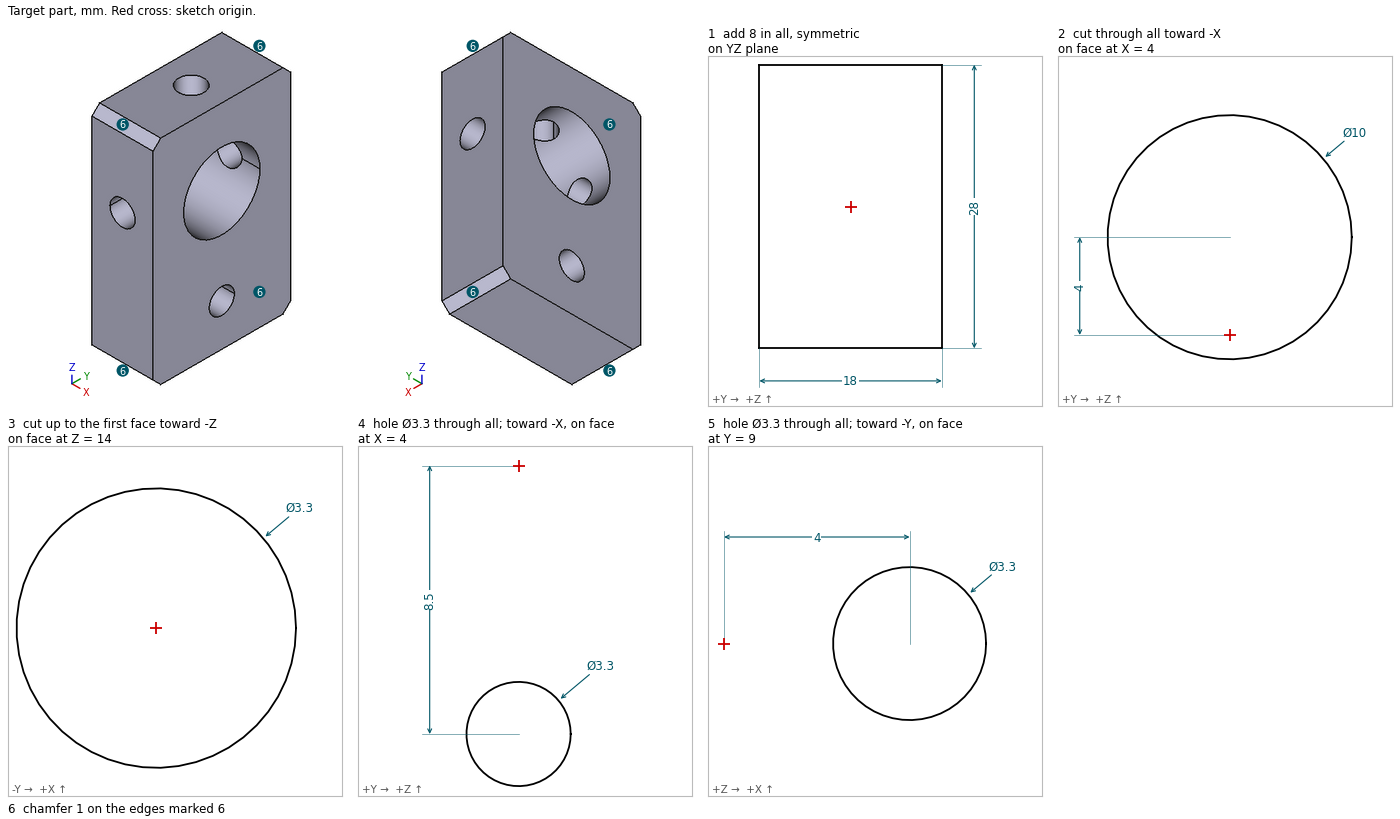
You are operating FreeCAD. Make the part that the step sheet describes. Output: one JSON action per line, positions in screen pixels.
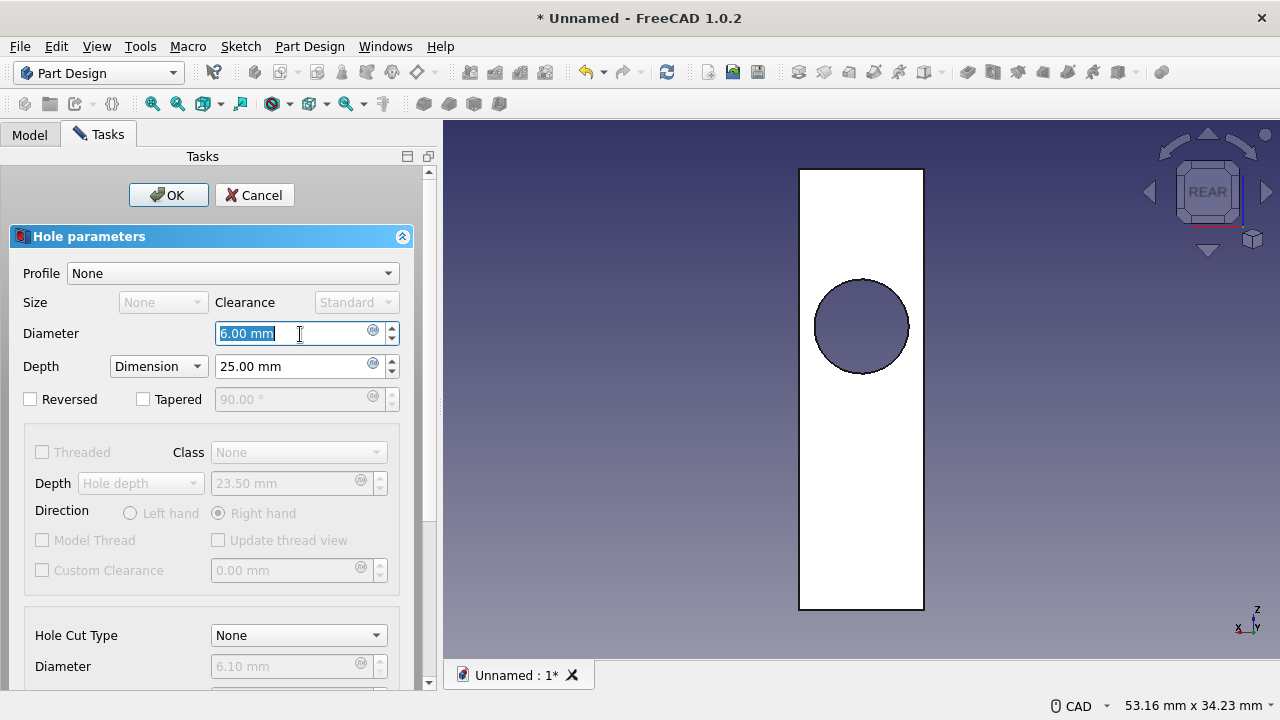
{"action": "type", "text": "3.3"}
{"action": "key", "text": "Tab"}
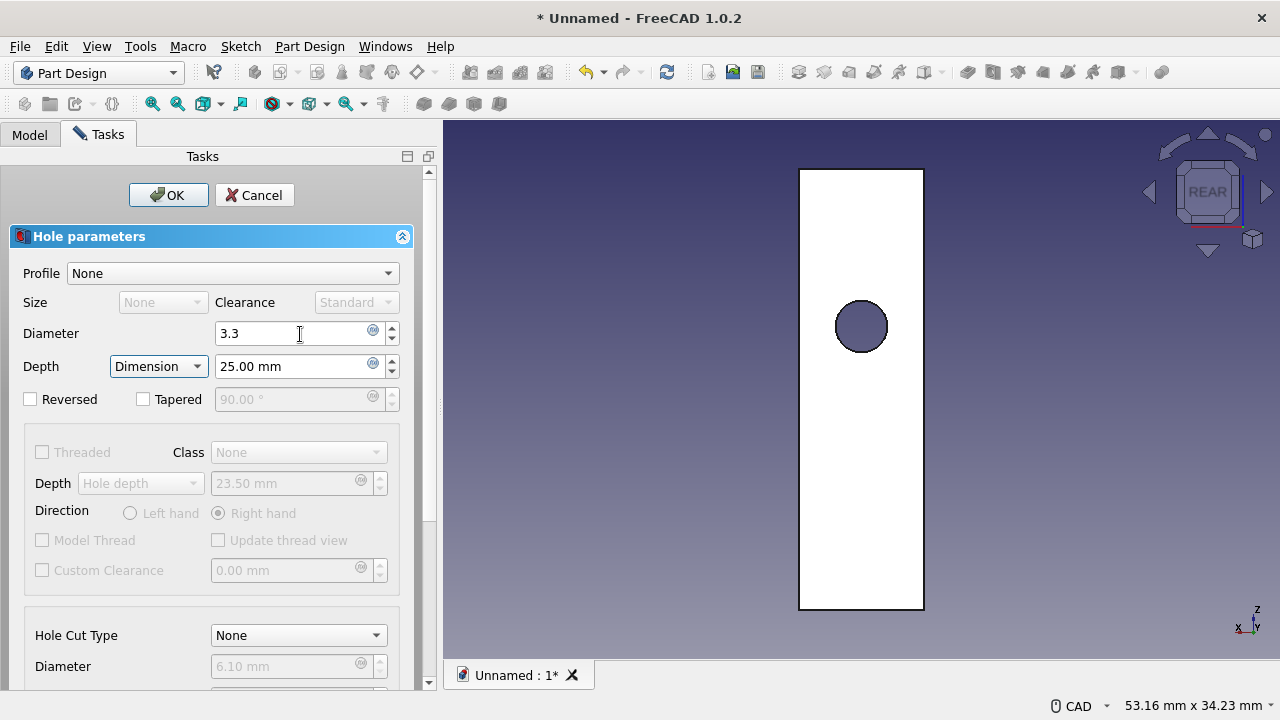
{"action": "left_click", "coordinate": [160, 366]}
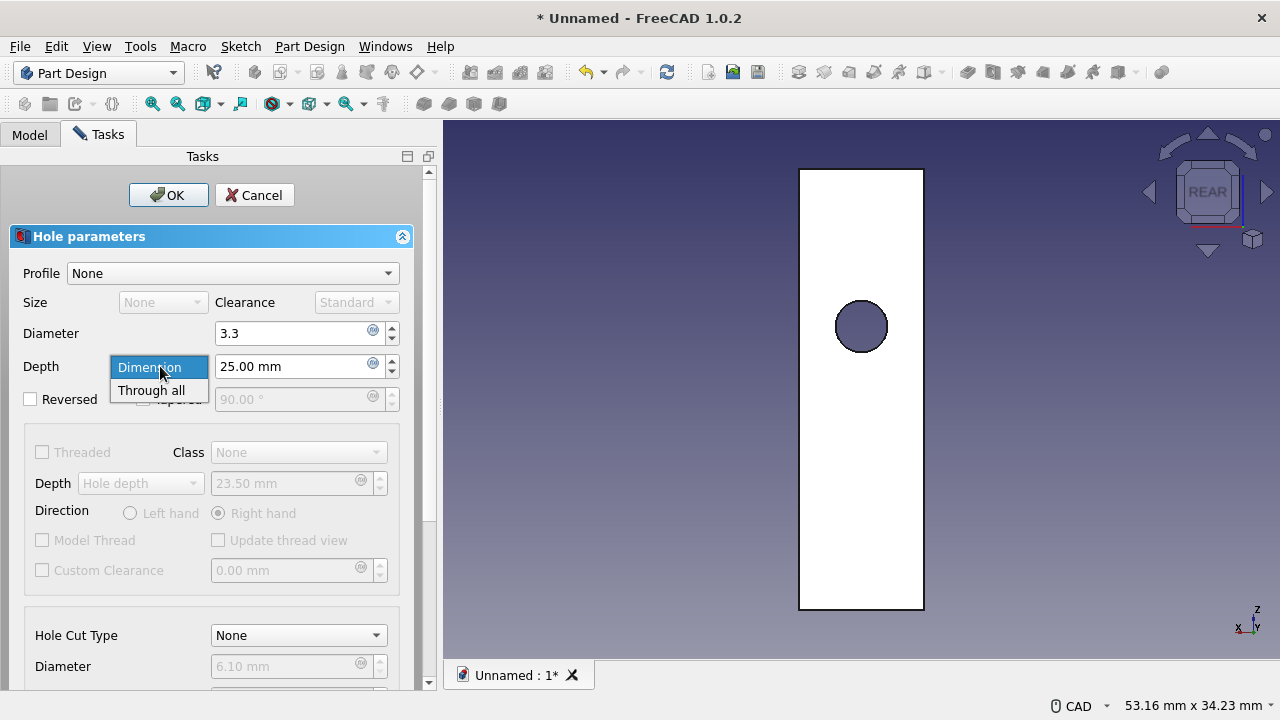
{"action": "left_click", "coordinate": [158, 390]}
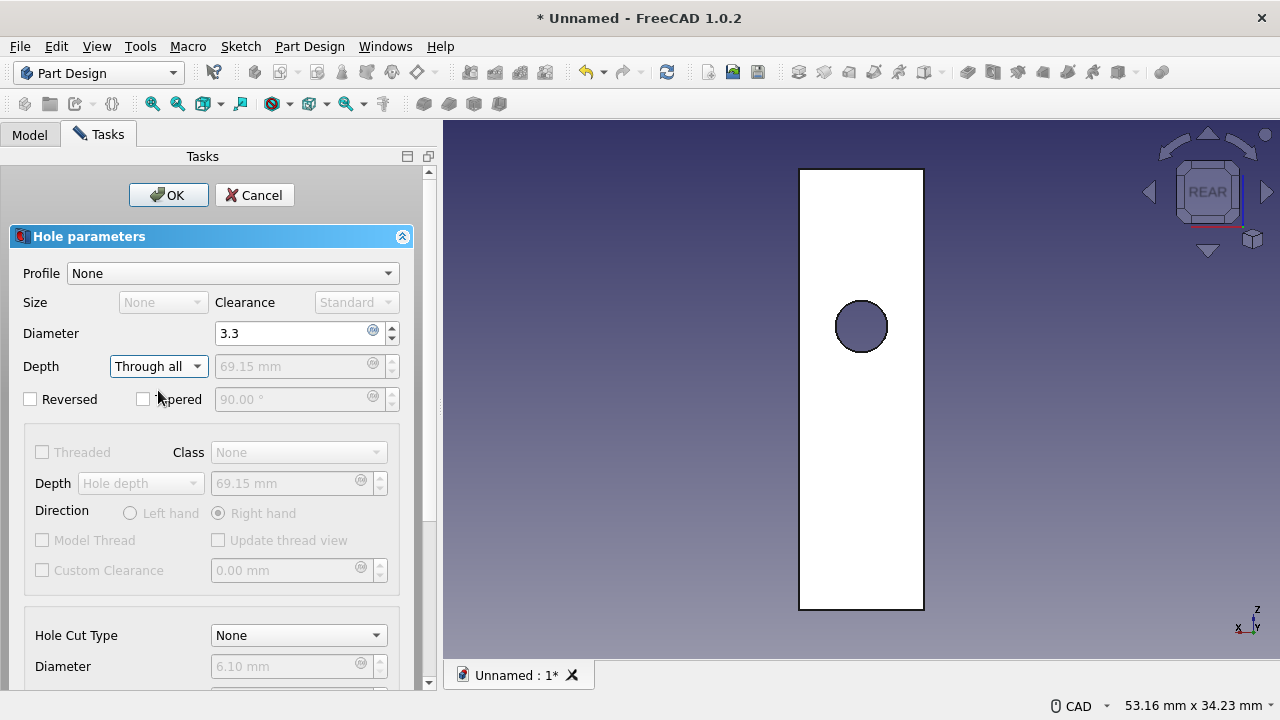
{"action": "left_click", "coordinate": [169, 195]}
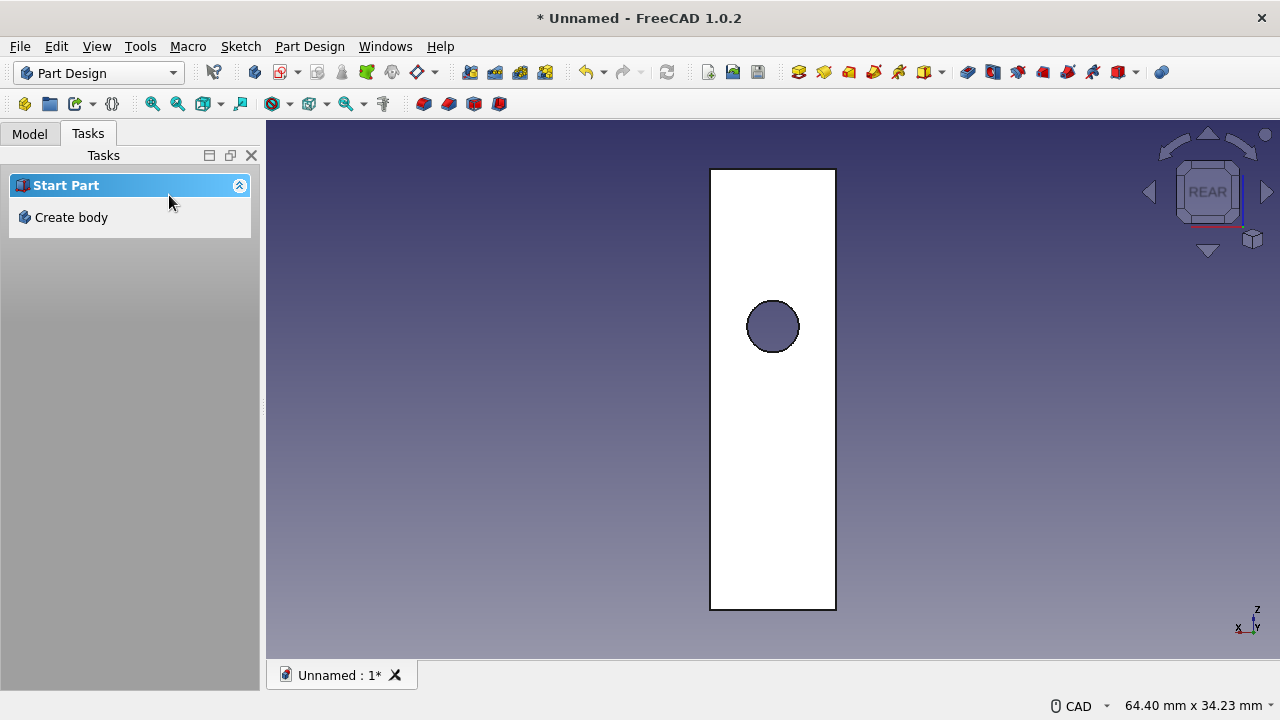
{"action": "left_click", "coordinate": [773, 168]}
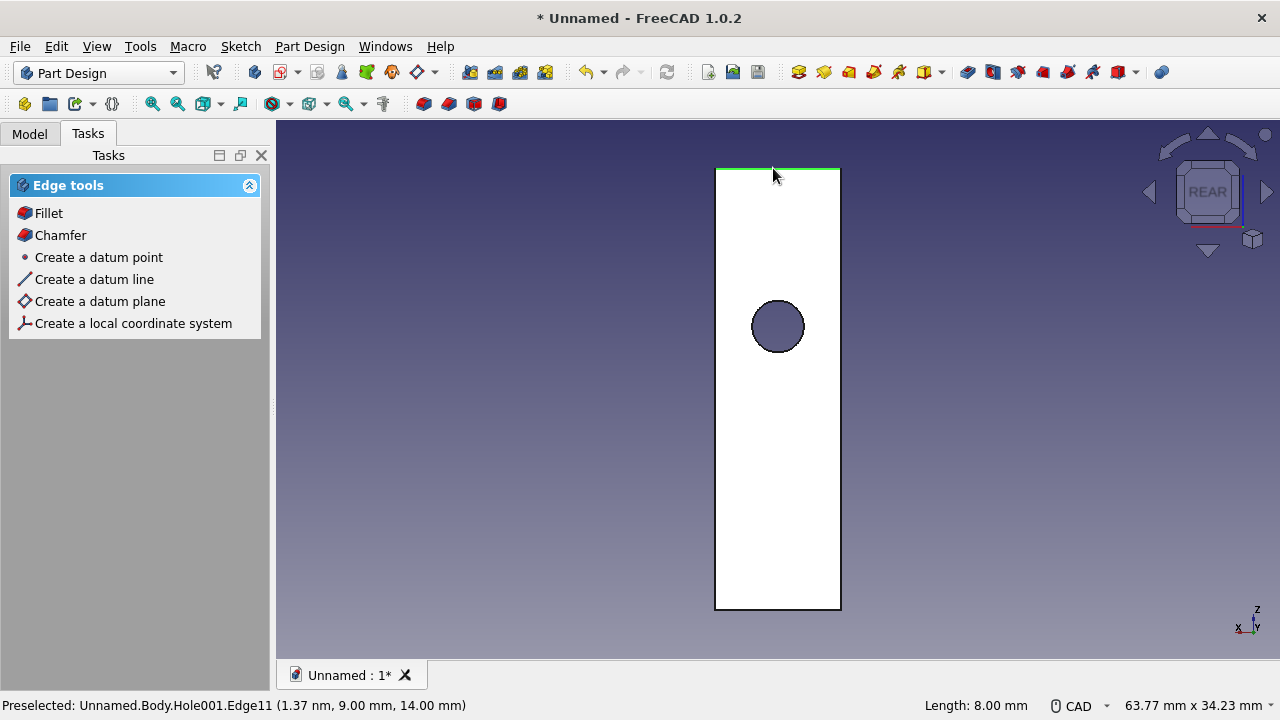
{"action": "left_click", "coordinate": [778, 609], "text": "ctrl"}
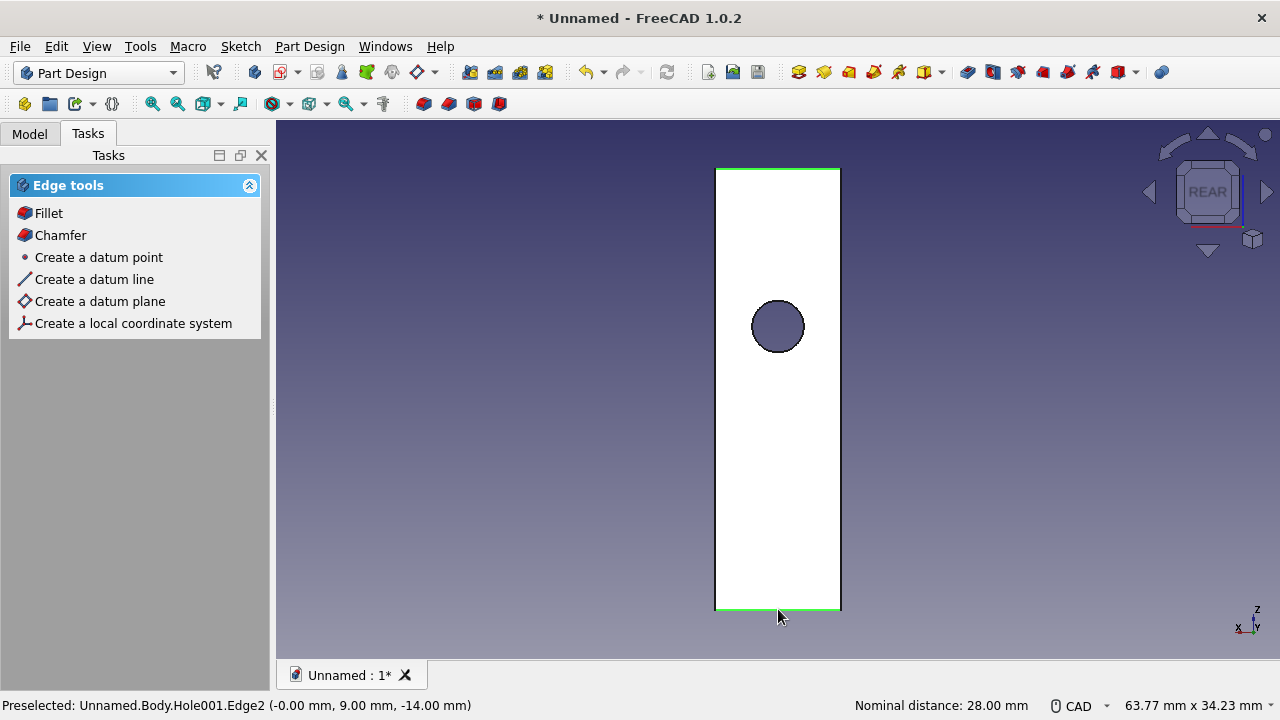
{"action": "key", "text": "0"}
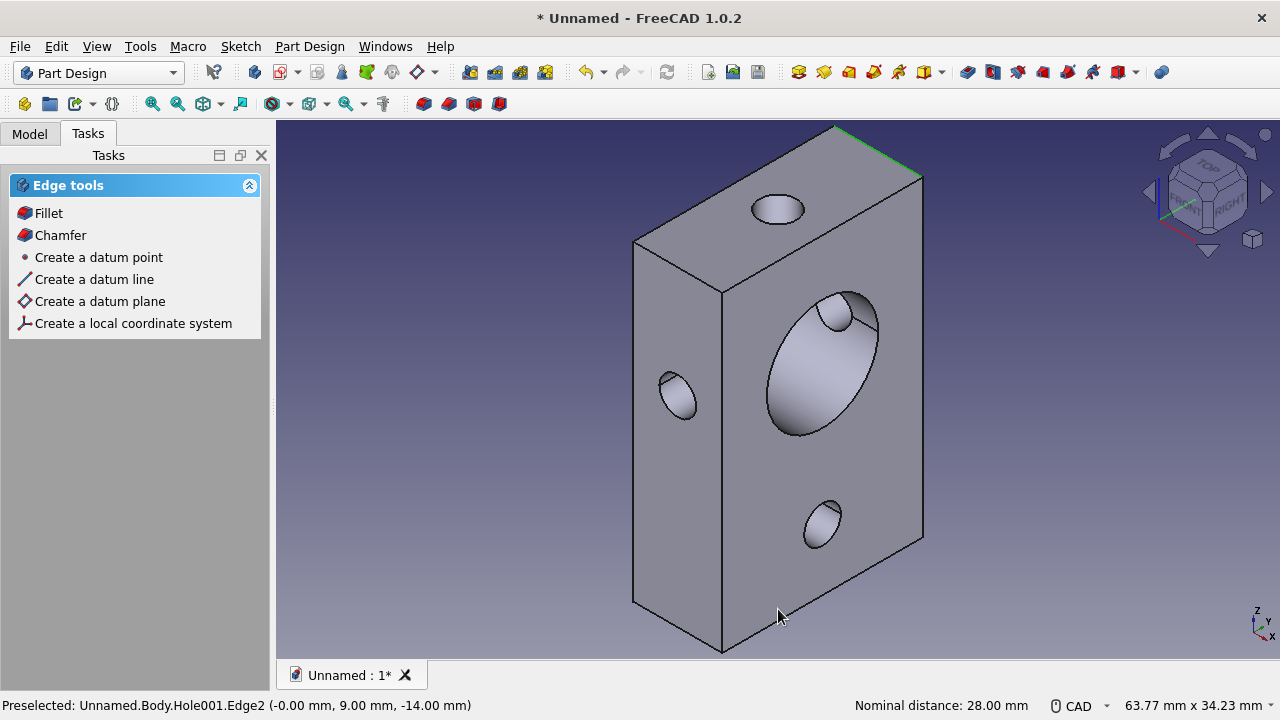
{"action": "left_click", "coordinate": [678, 266], "text": "ctrl"}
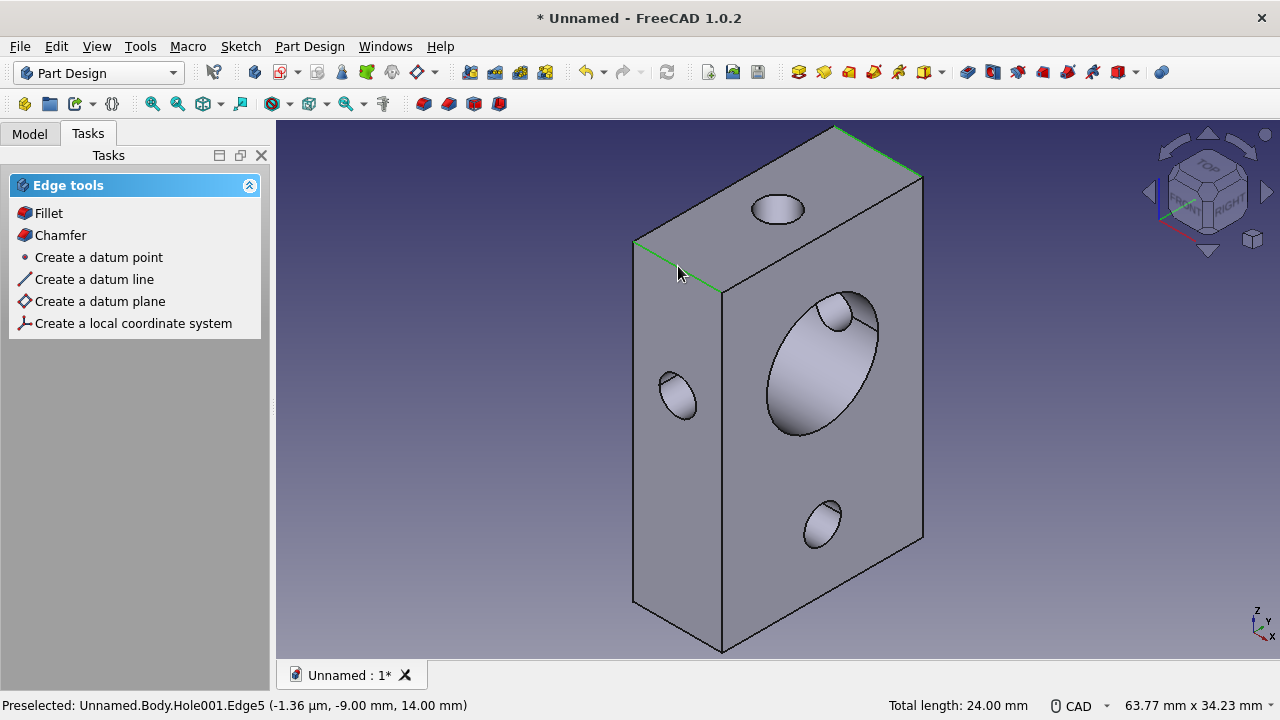
{"action": "key", "text": "2"}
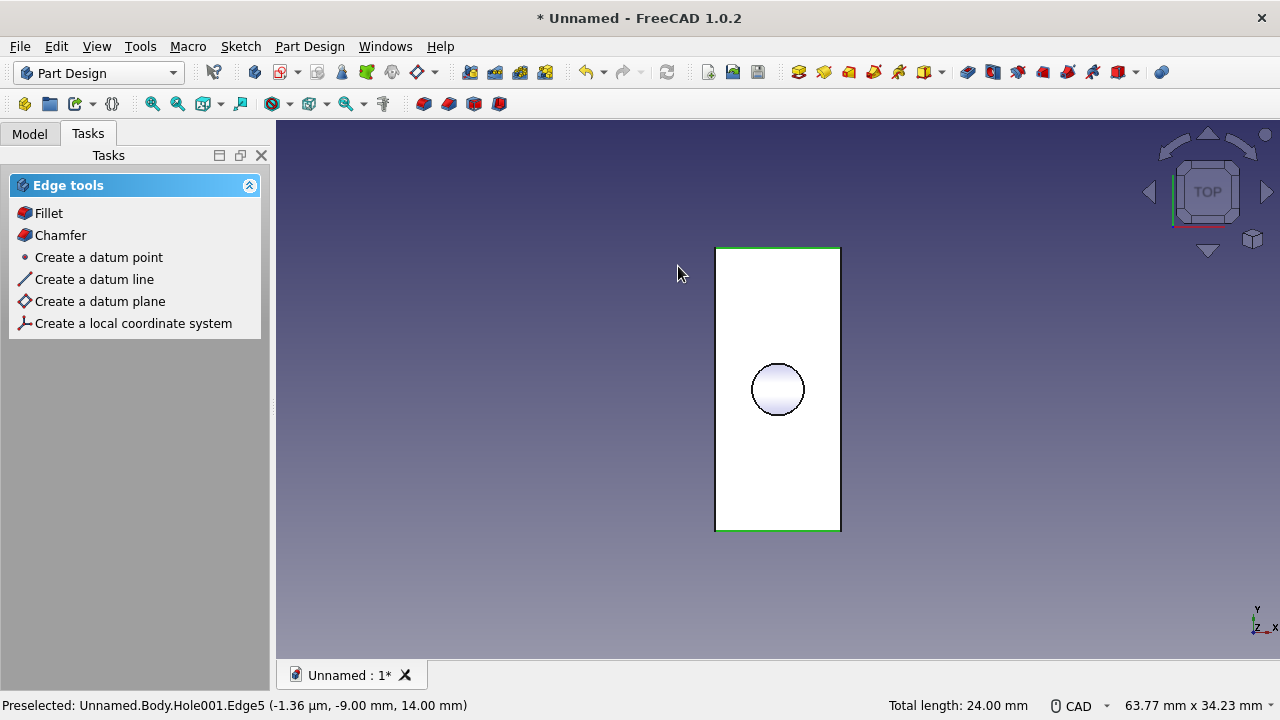
{"action": "key", "text": "1"}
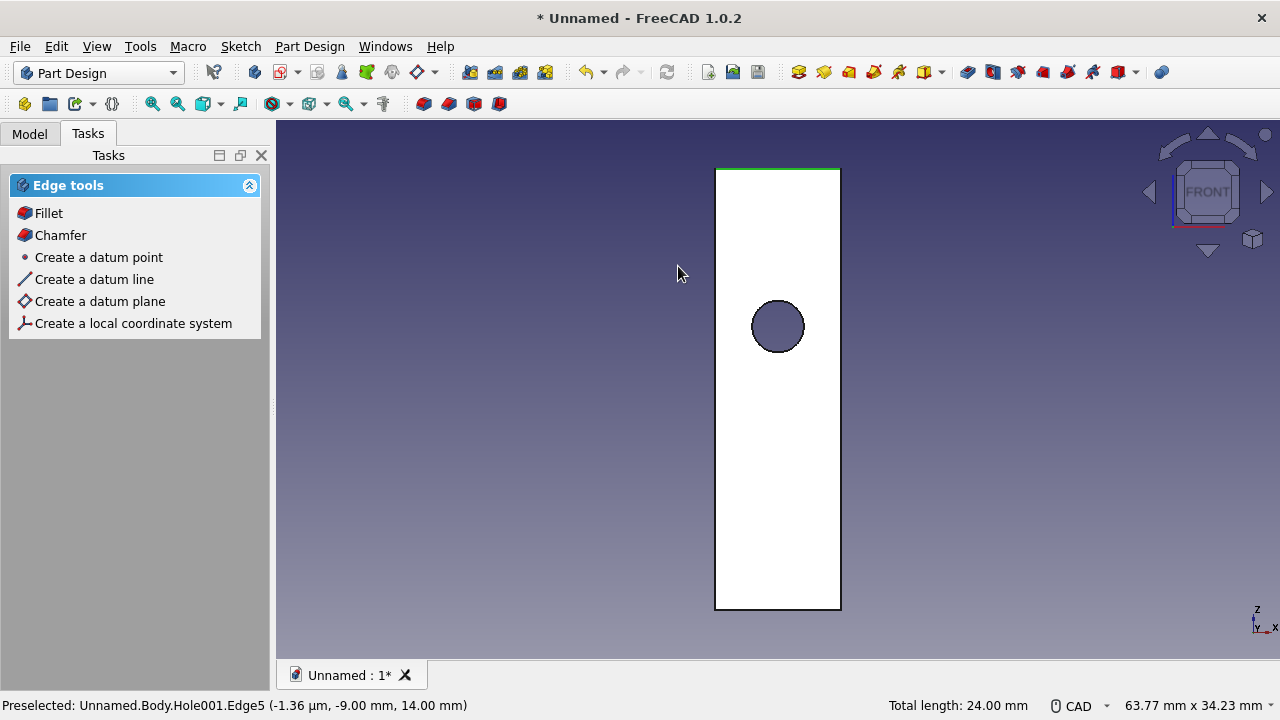
{"action": "left_click", "coordinate": [778, 609], "text": "ctrl"}